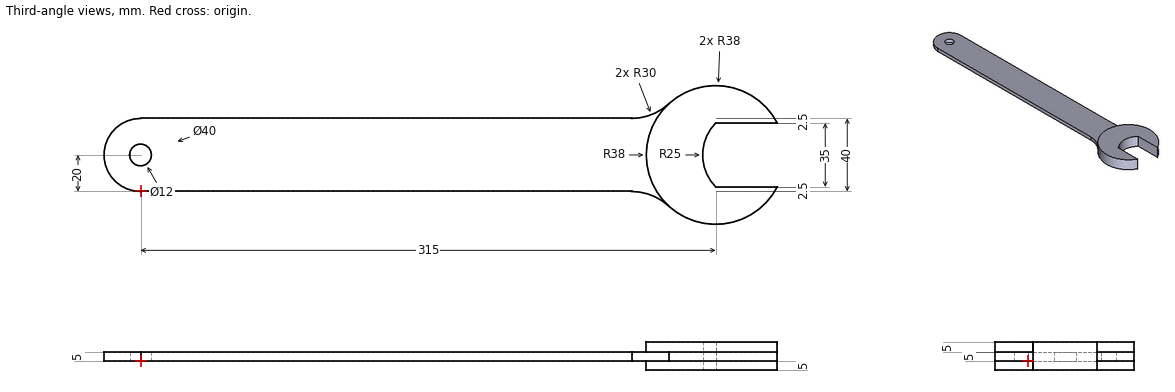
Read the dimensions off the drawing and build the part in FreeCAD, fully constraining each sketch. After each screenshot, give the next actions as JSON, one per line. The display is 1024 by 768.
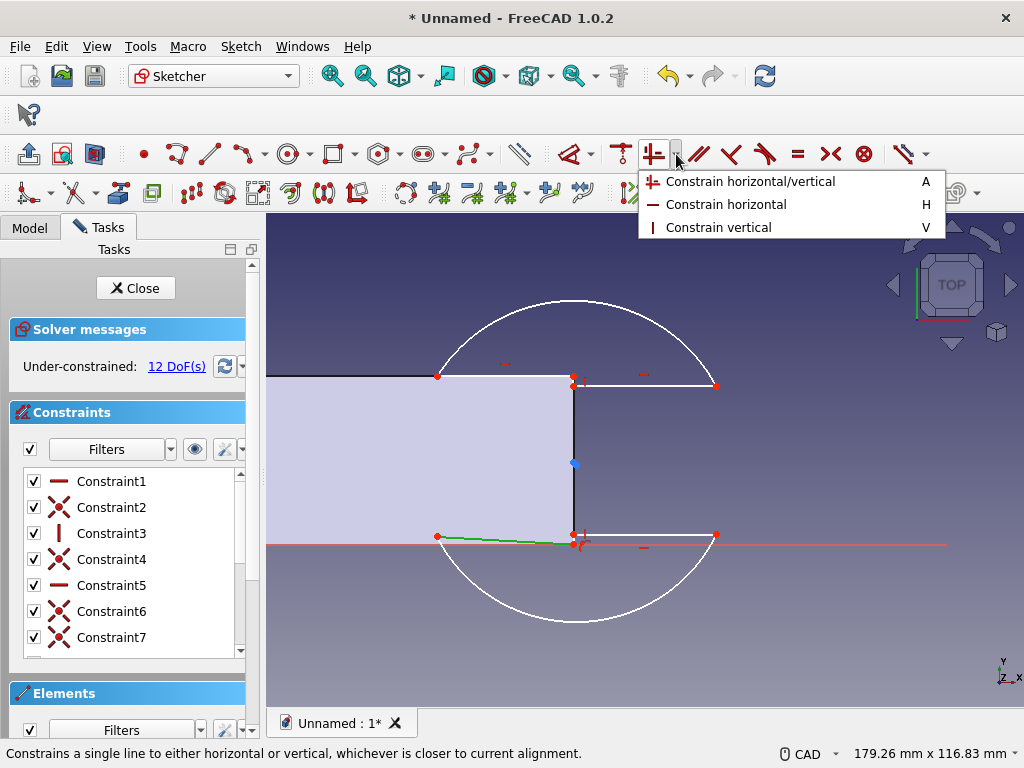
{"action": "left_click", "coordinate": [792, 204]}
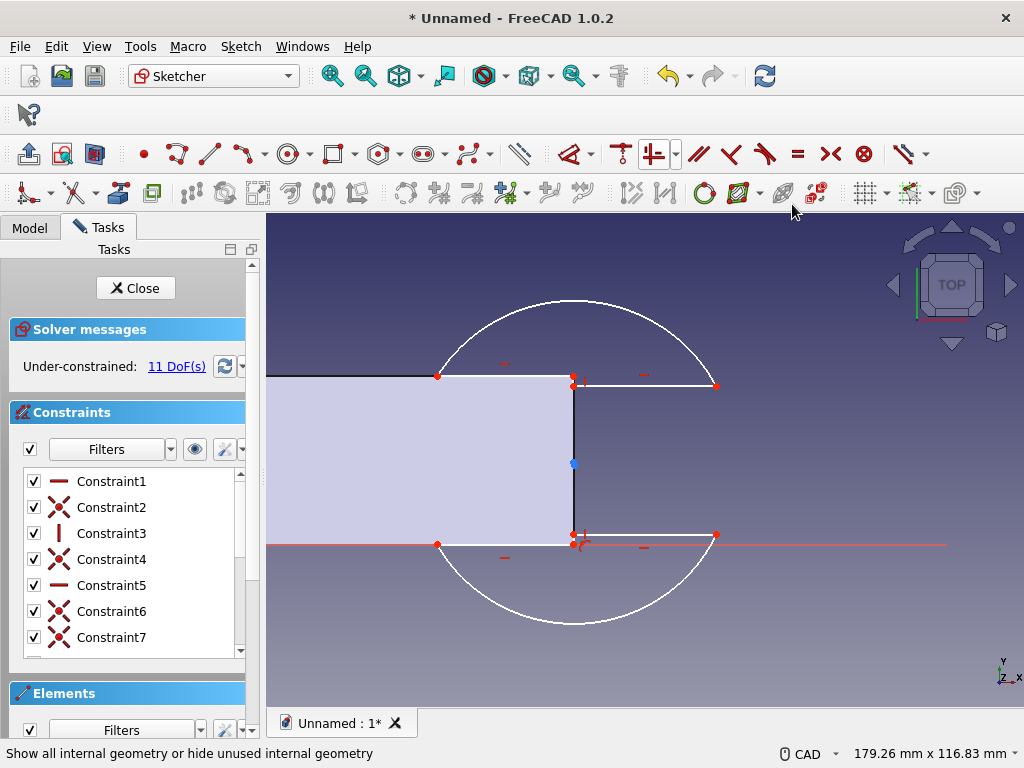
{"action": "left_click", "coordinate": [645, 317]}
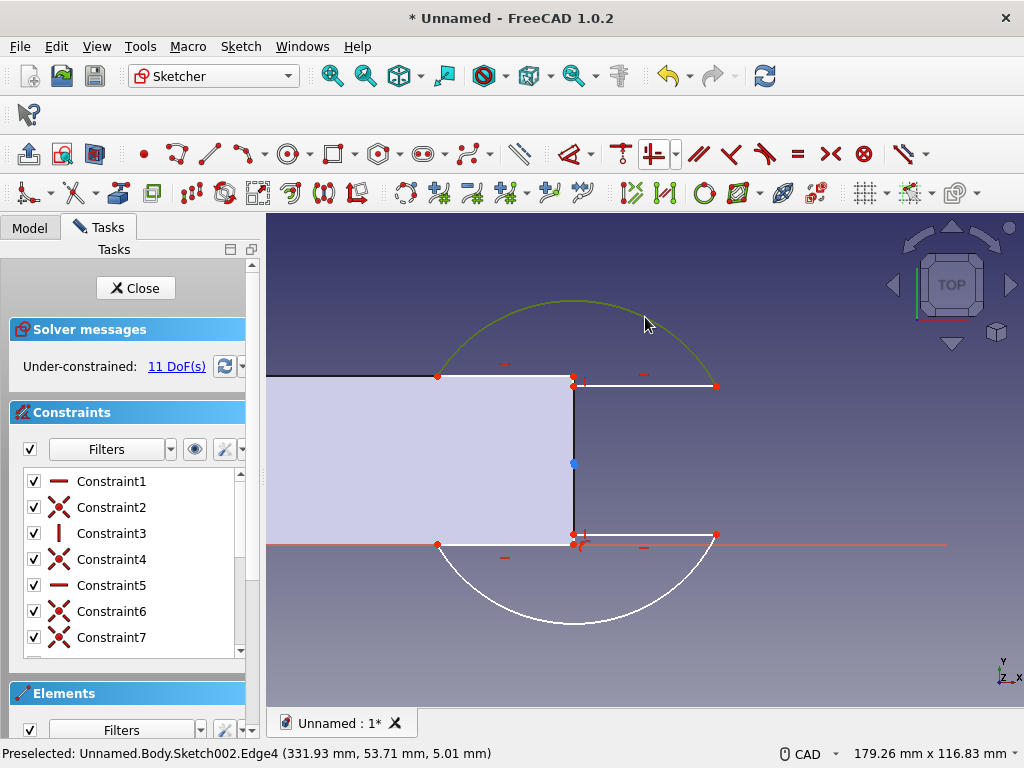
{"action": "left_click", "coordinate": [513, 612]}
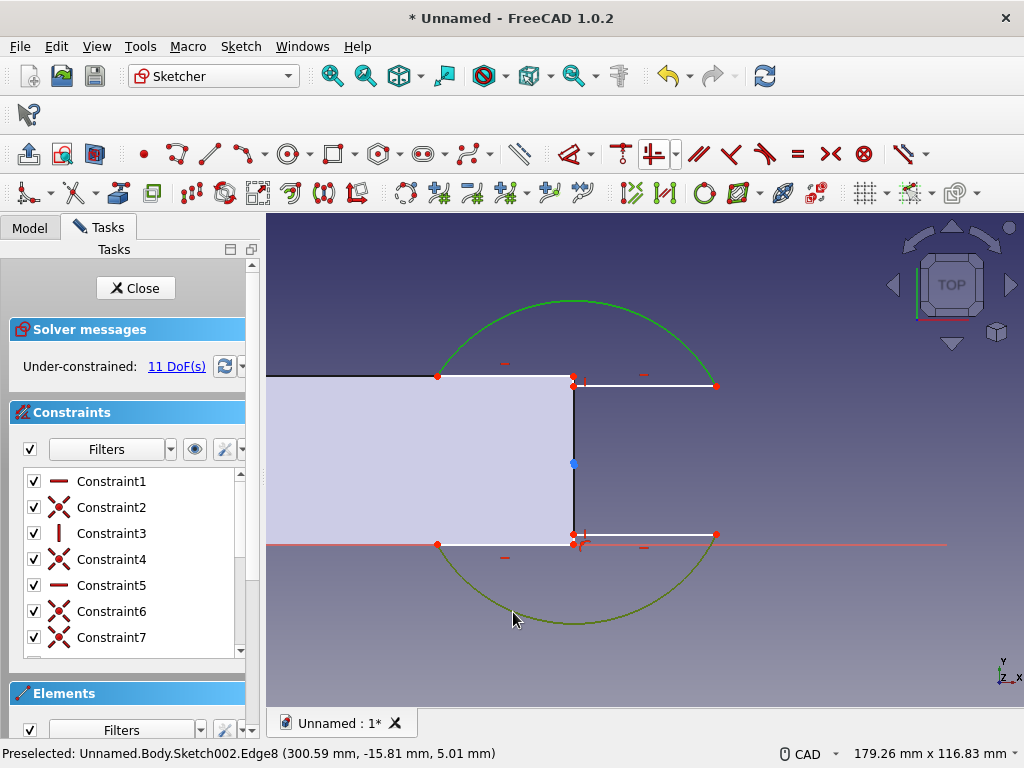
{"action": "left_click", "coordinate": [621, 154]}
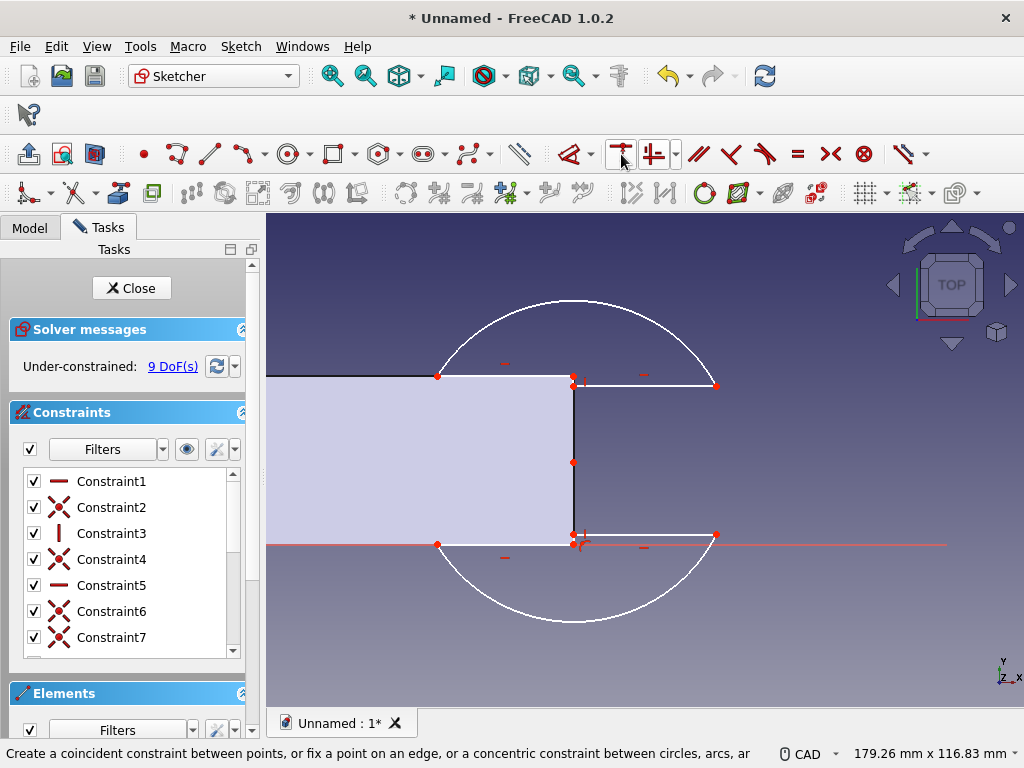
{"action": "left_click", "coordinate": [645, 317]}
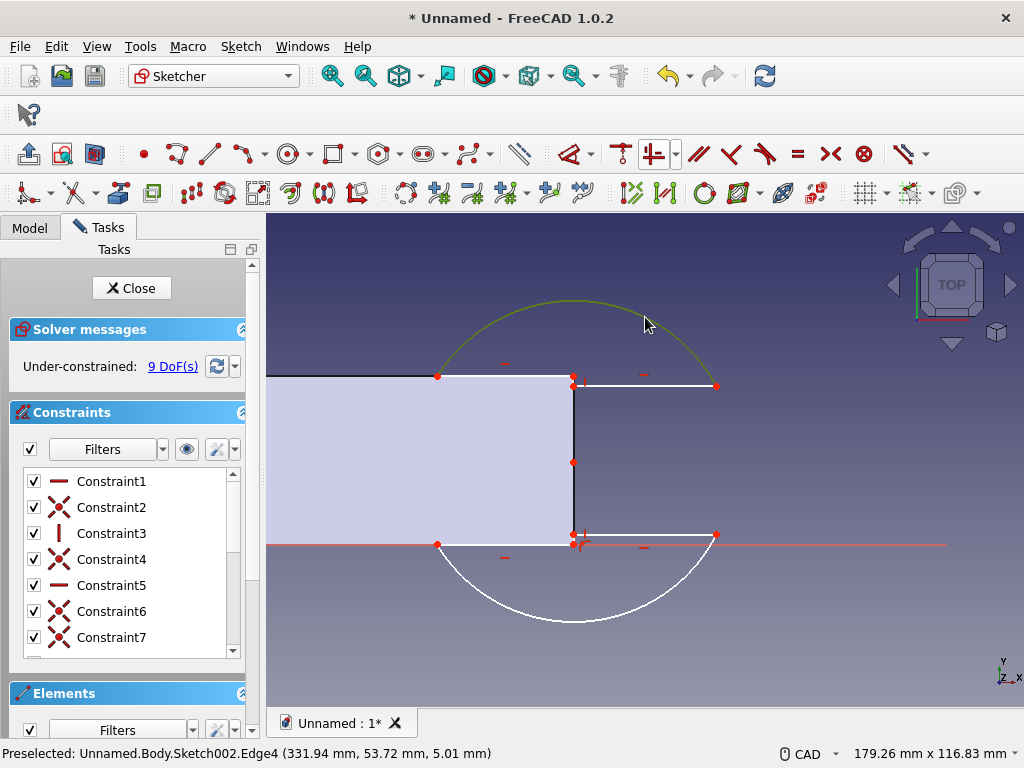
{"action": "left_click", "coordinate": [513, 610]}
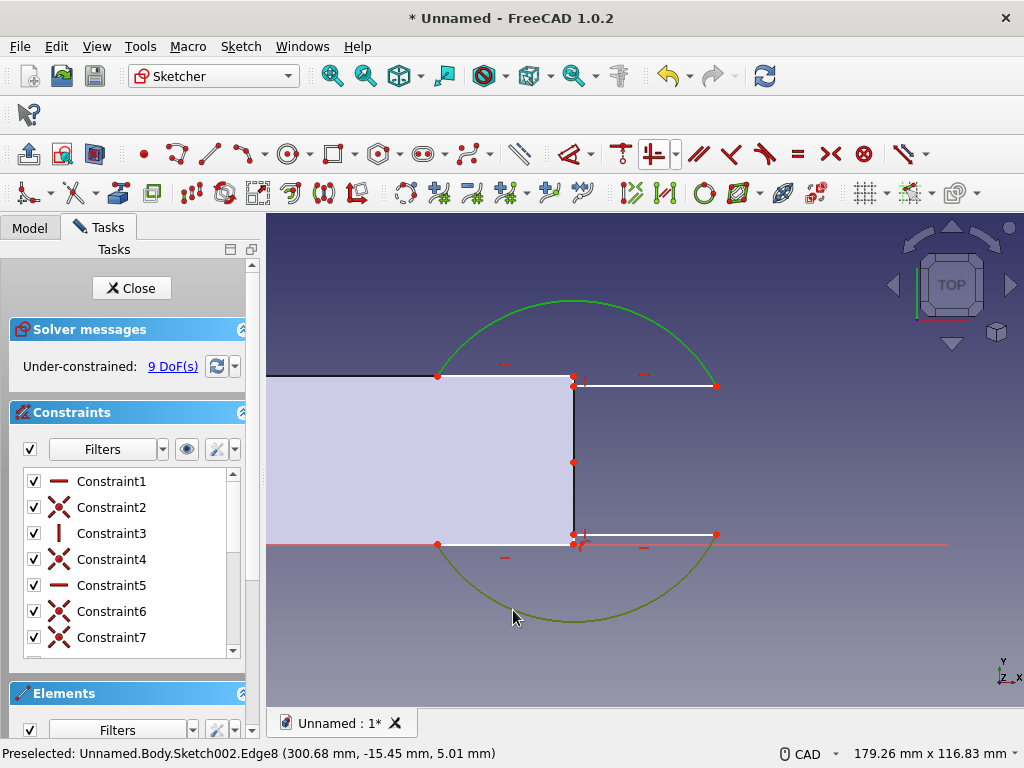
{"action": "left_click", "coordinate": [798, 154]}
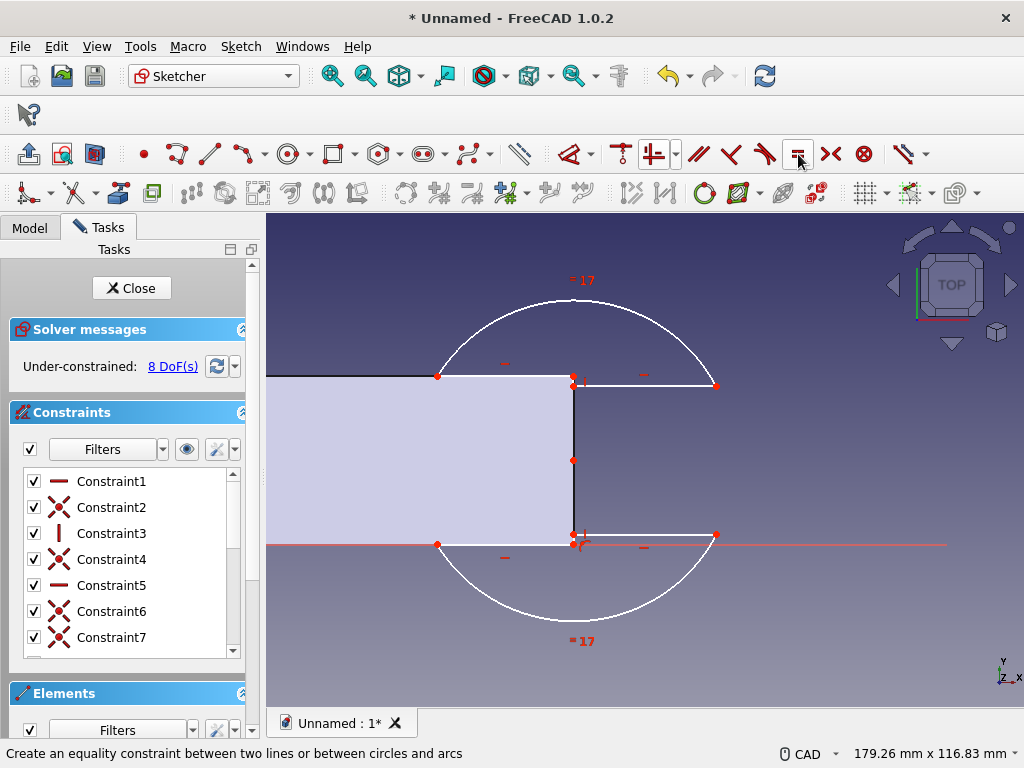
{"action": "left_click", "coordinate": [568, 154]}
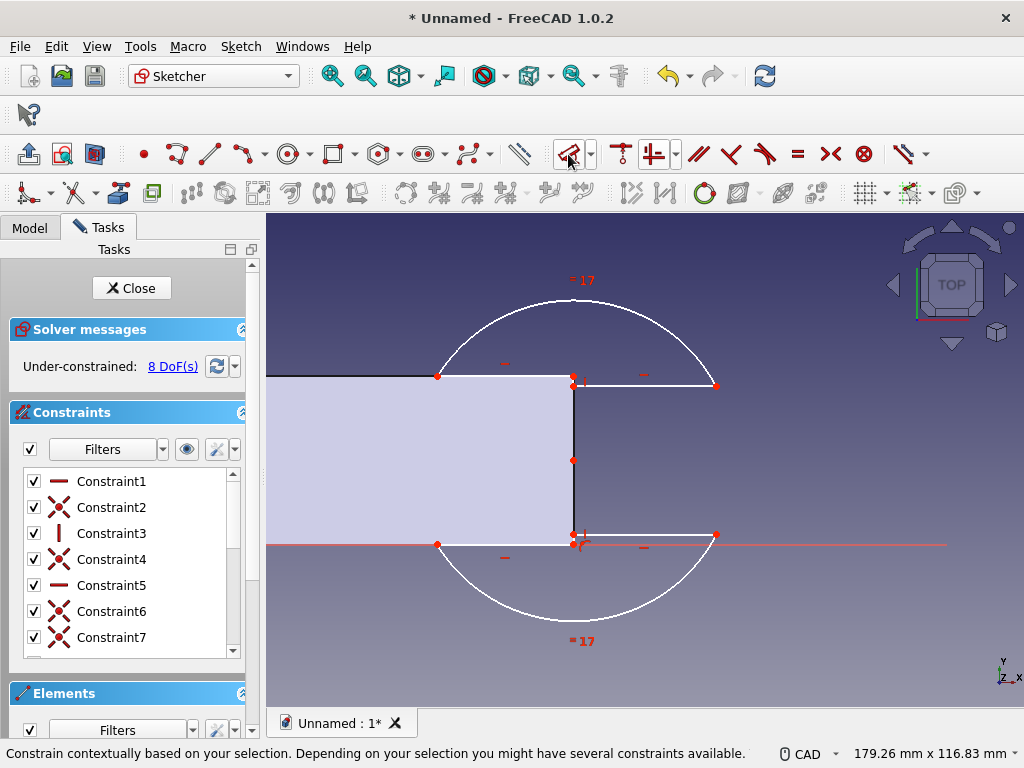
{"action": "left_click", "coordinate": [645, 317]}
{"action": "left_click", "coordinate": [659, 288]}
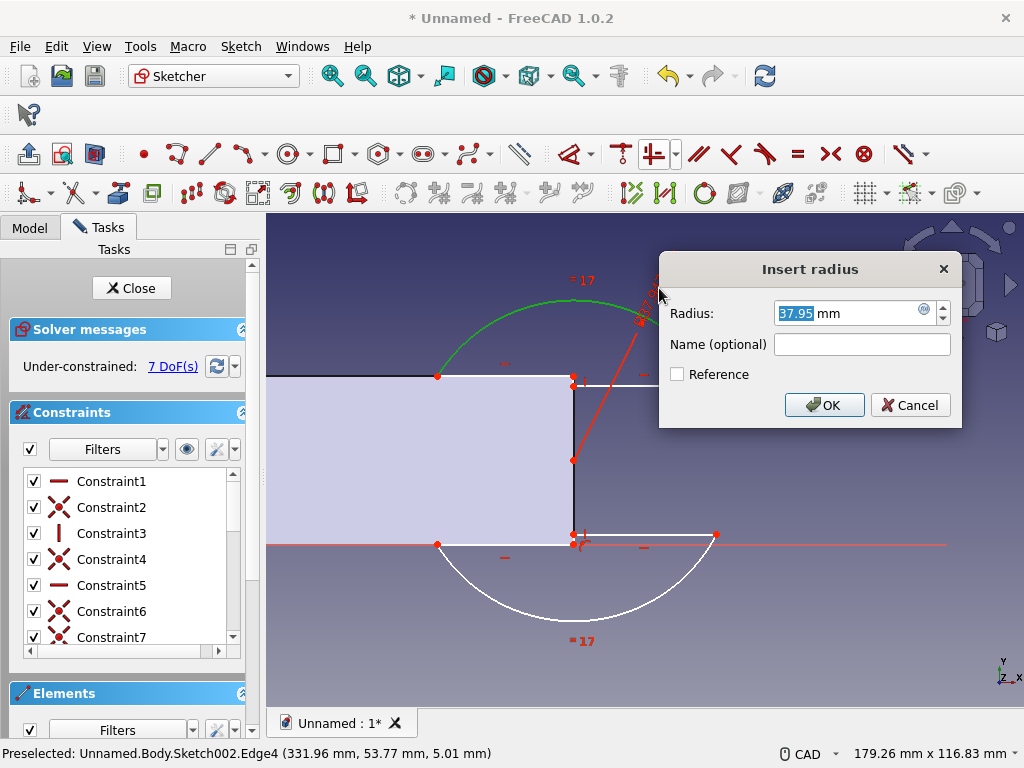
{"action": "type", "text": "38"}
{"action": "key", "text": "Return"}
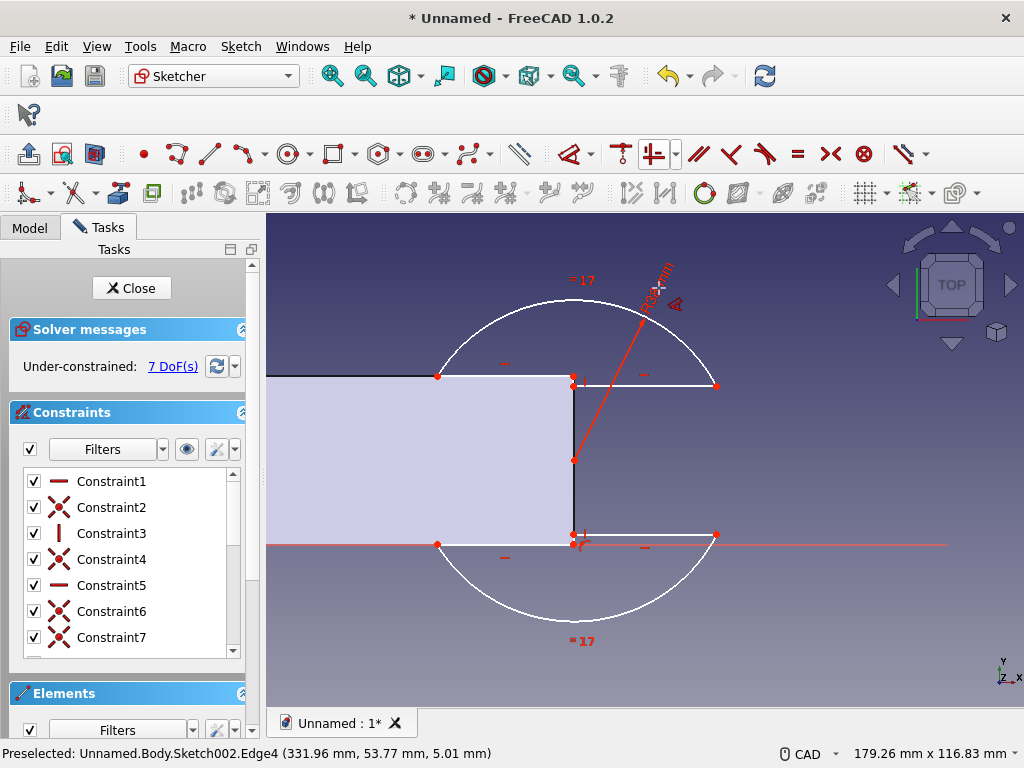
{"action": "scroll", "coordinate": [573, 381], "scroll_direction": "up", "scroll_amount": 7}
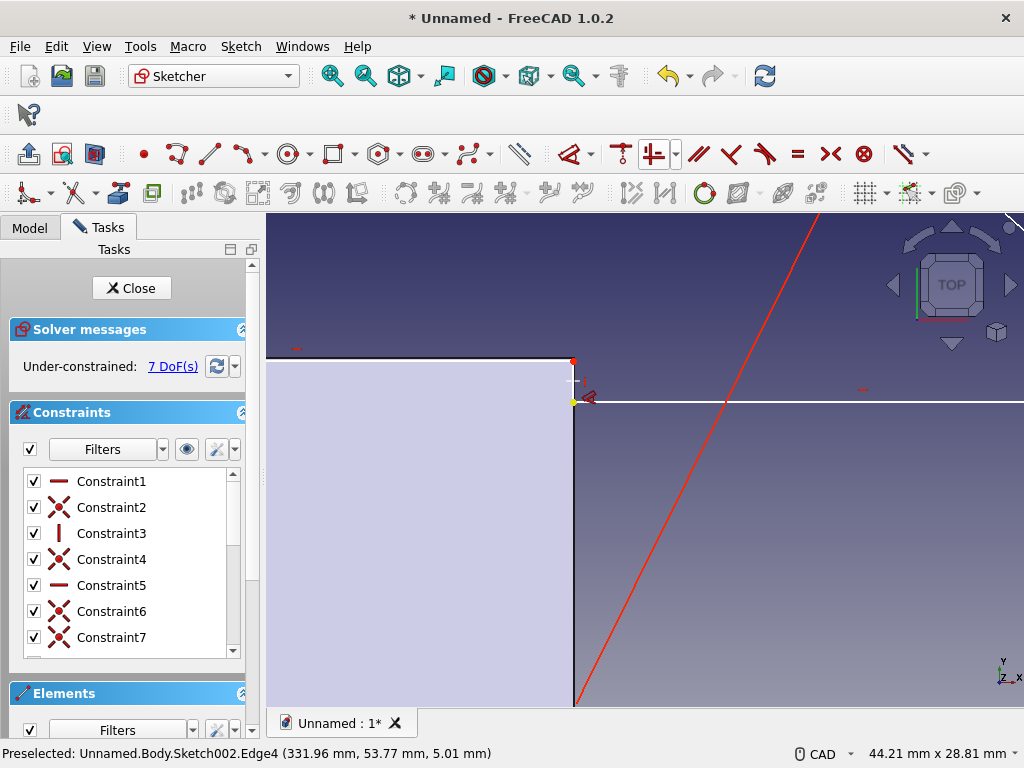
{"action": "left_click", "coordinate": [573, 382]}
{"action": "left_click", "coordinate": [539, 382]}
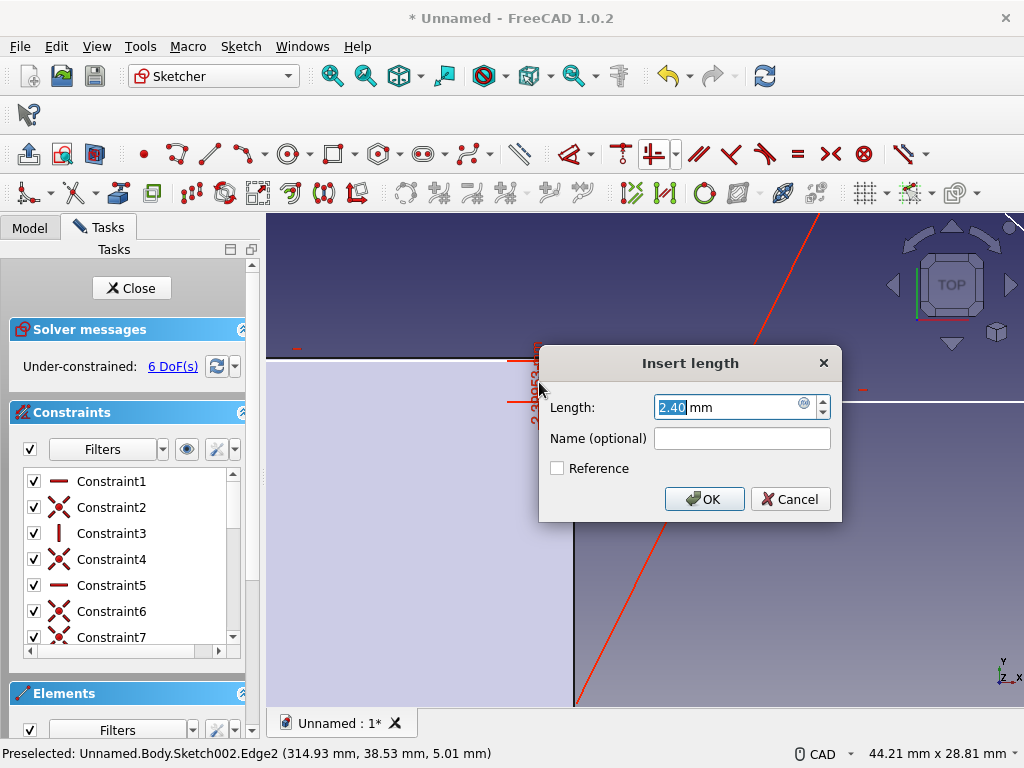
{"action": "type", "text": "2.5"}
{"action": "key", "text": "Return"}